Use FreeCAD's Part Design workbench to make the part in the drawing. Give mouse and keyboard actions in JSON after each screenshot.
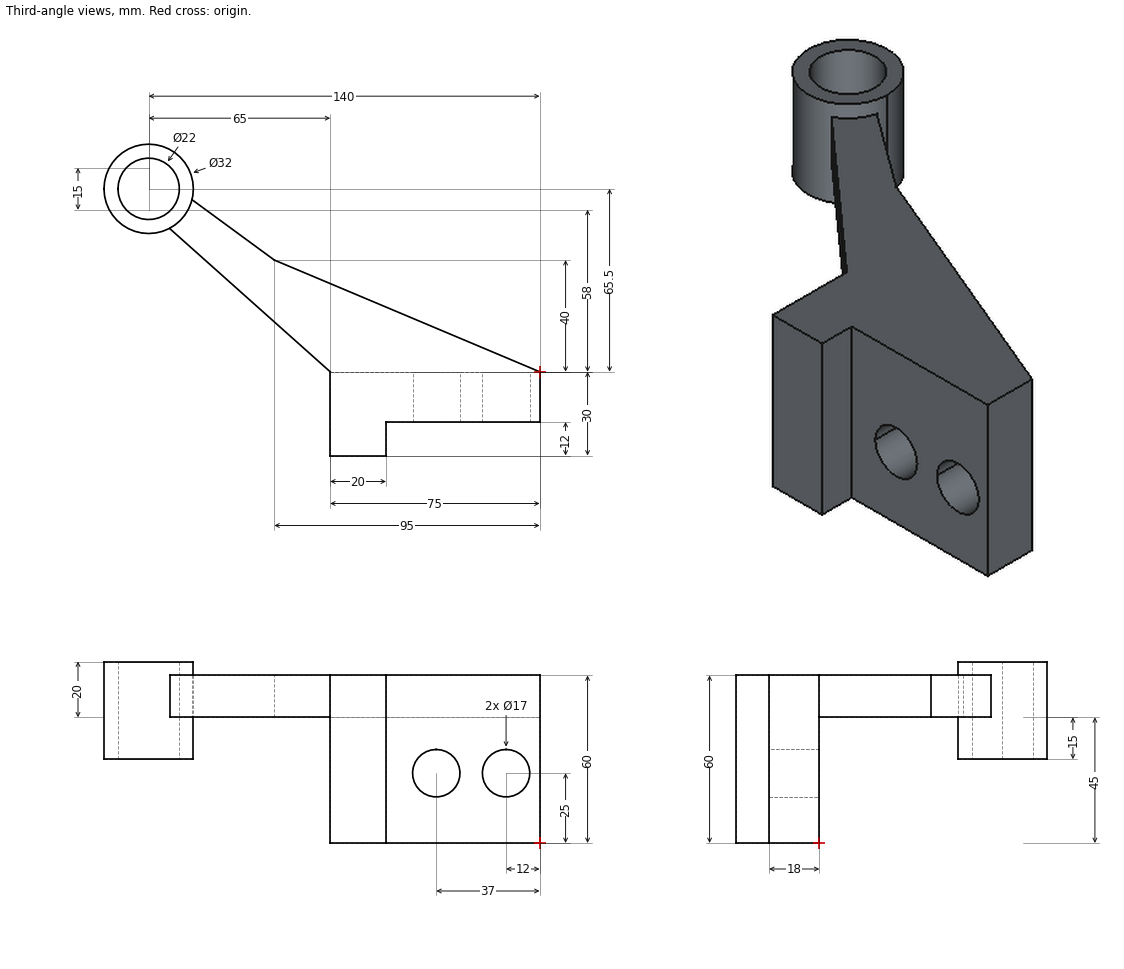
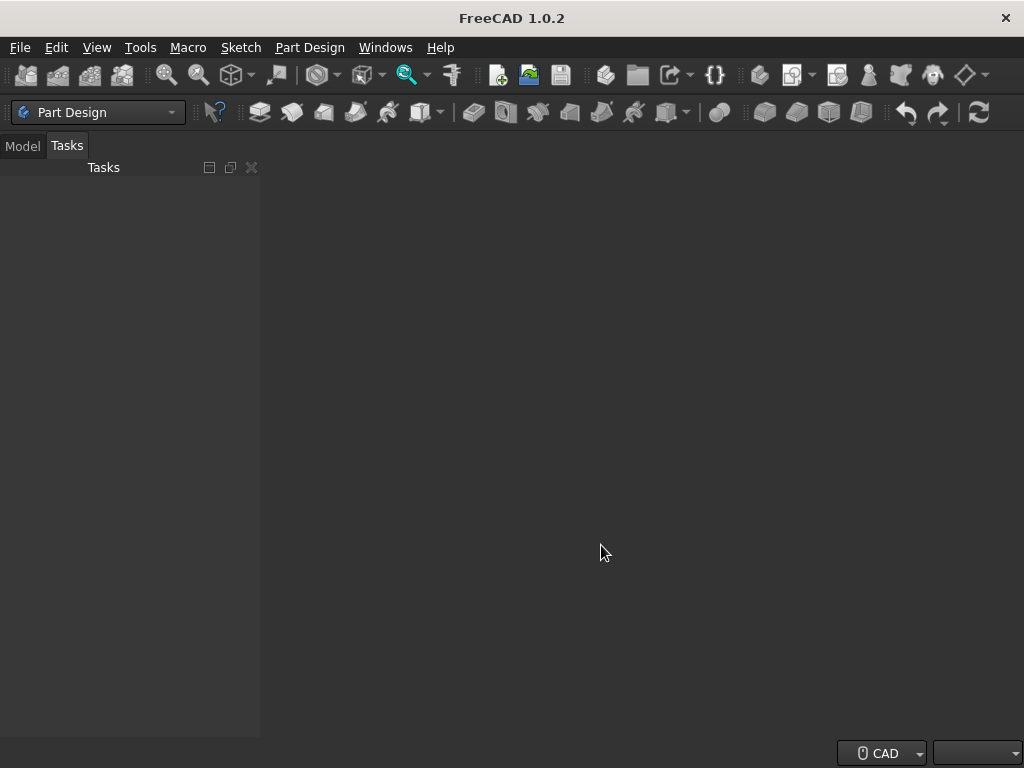
{"action": "left_click", "coordinate": [498, 76]}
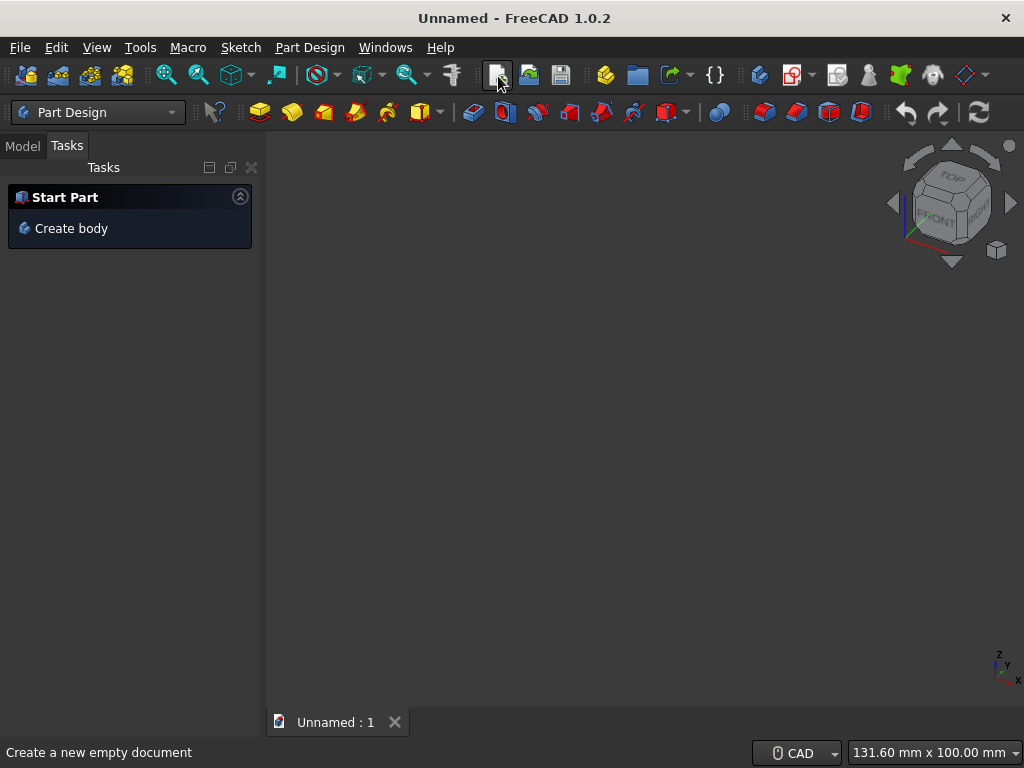
{"action": "left_click", "coordinate": [792, 76]}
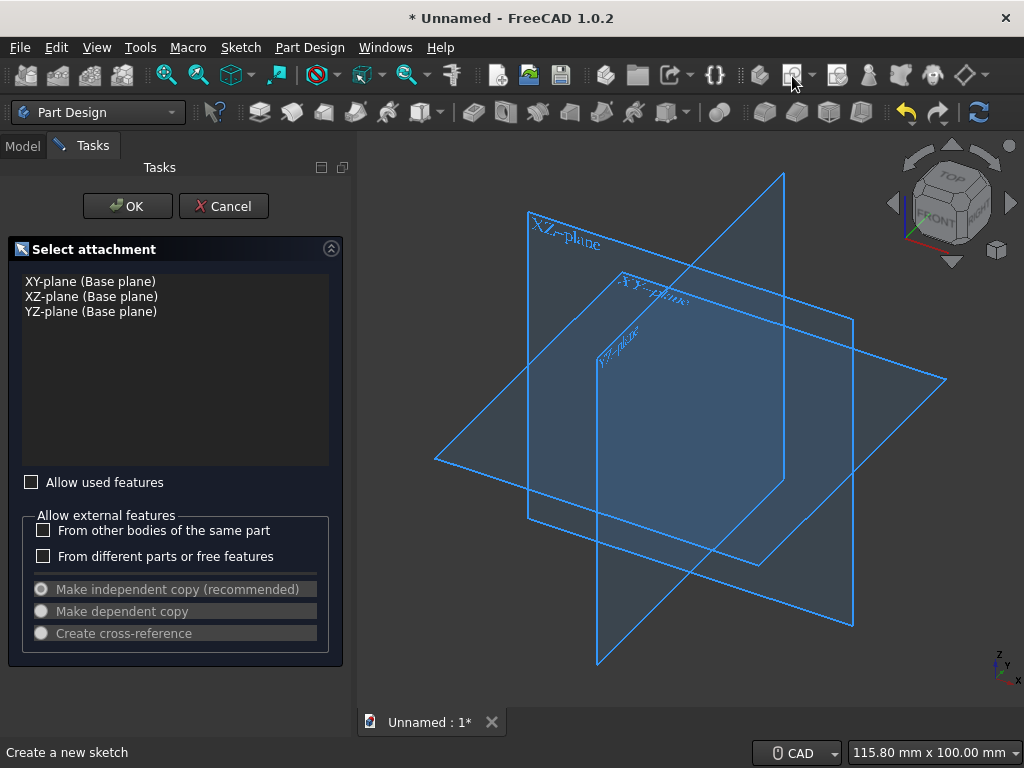
{"action": "left_click", "coordinate": [82, 282]}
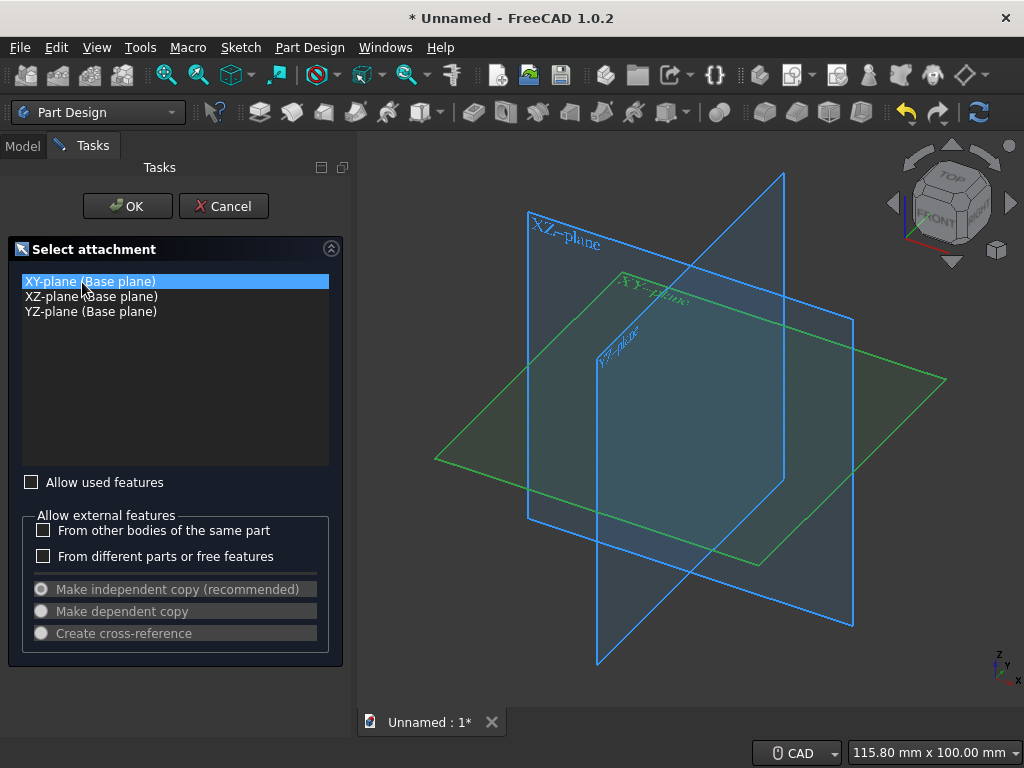
{"action": "left_click", "coordinate": [128, 206]}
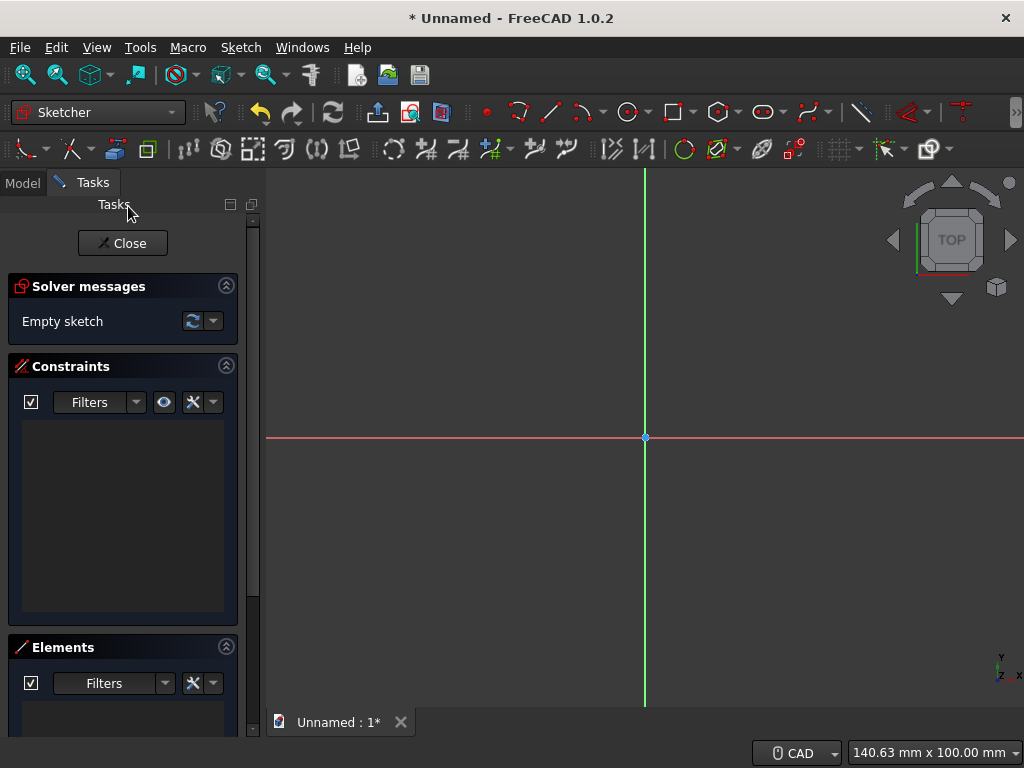
{"action": "scroll", "coordinate": [859, 196], "scroll_direction": "down", "scroll_amount": 1}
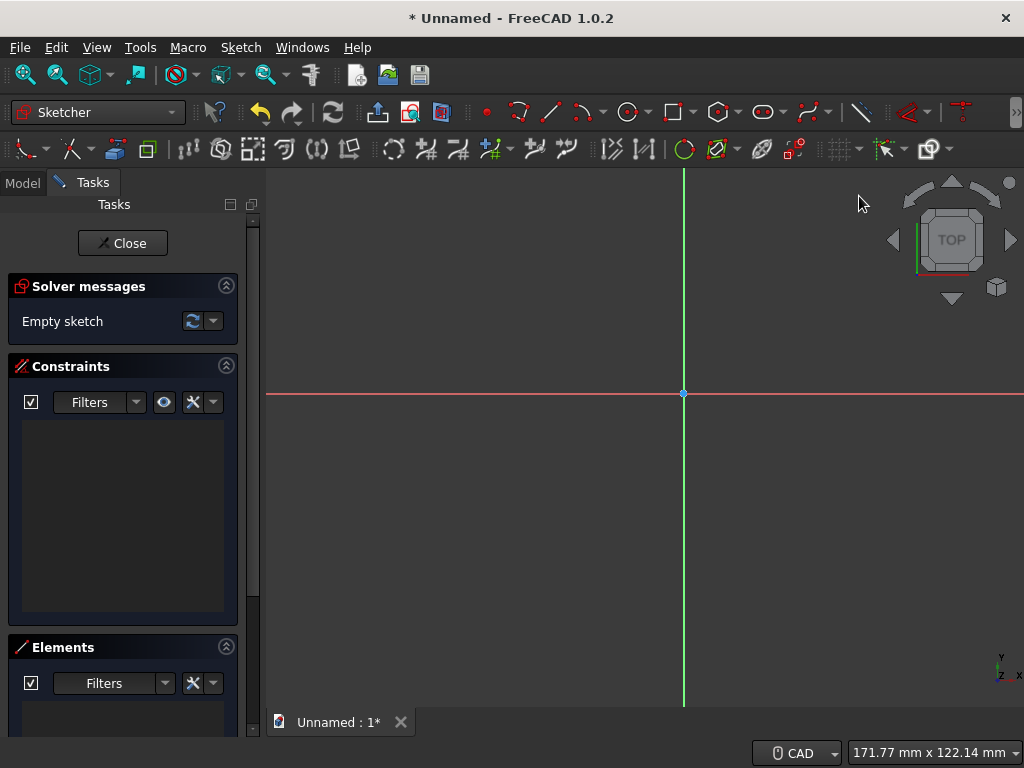
{"action": "left_click", "coordinate": [520, 112]}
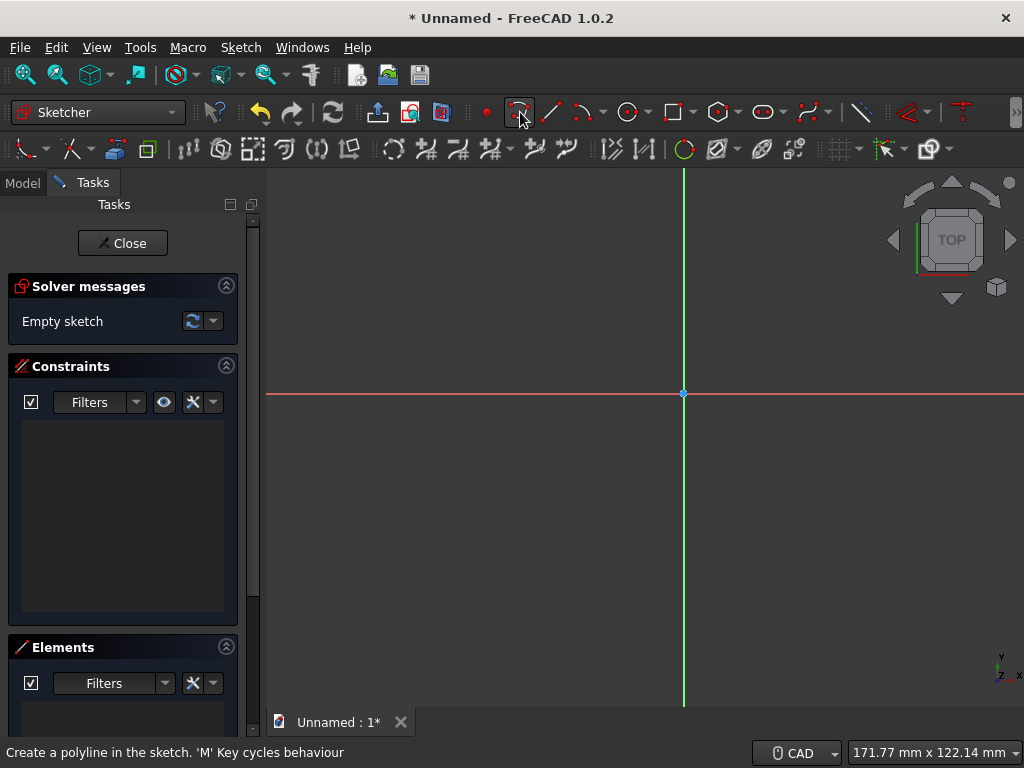
{"action": "left_click", "coordinate": [684, 394]}
{"action": "left_click", "coordinate": [353, 403]}
{"action": "left_click", "coordinate": [353, 526]}
{"action": "left_click", "coordinate": [441, 526]}
{"action": "left_click", "coordinate": [441, 473]}
{"action": "left_click", "coordinate": [675, 473]}
{"action": "left_click", "coordinate": [684, 394]}
{"action": "key", "text": "Escape"}
{"action": "key", "text": "Escape"}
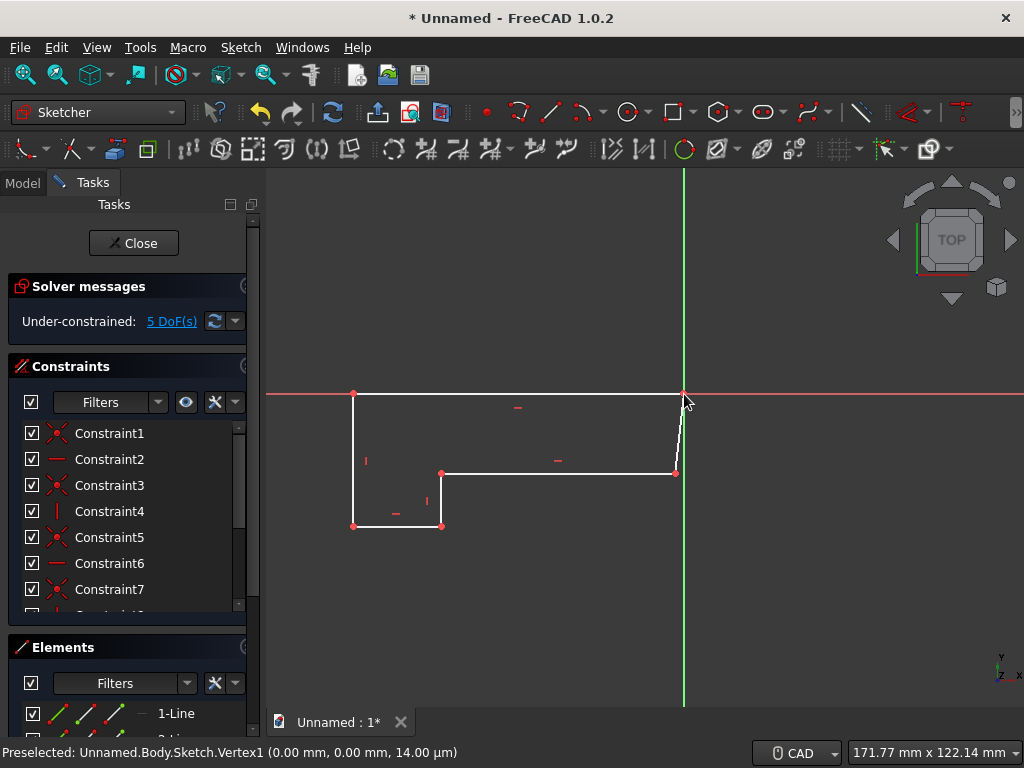
{"action": "left_click", "coordinate": [681, 418]}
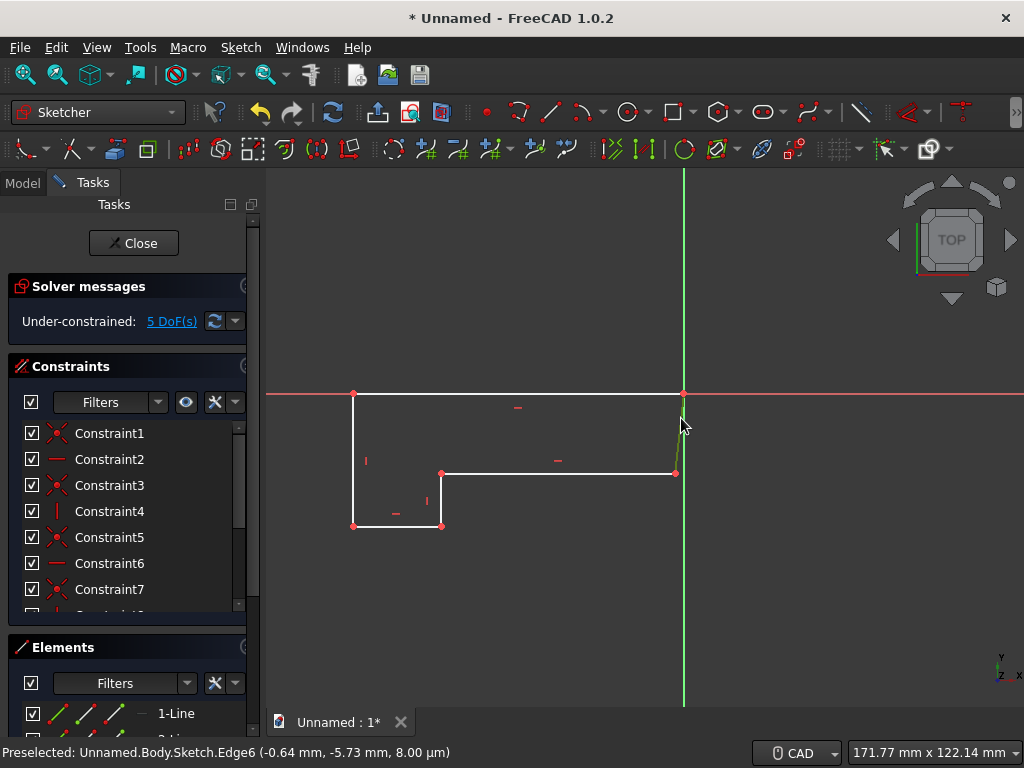
{"action": "key", "text": "v"}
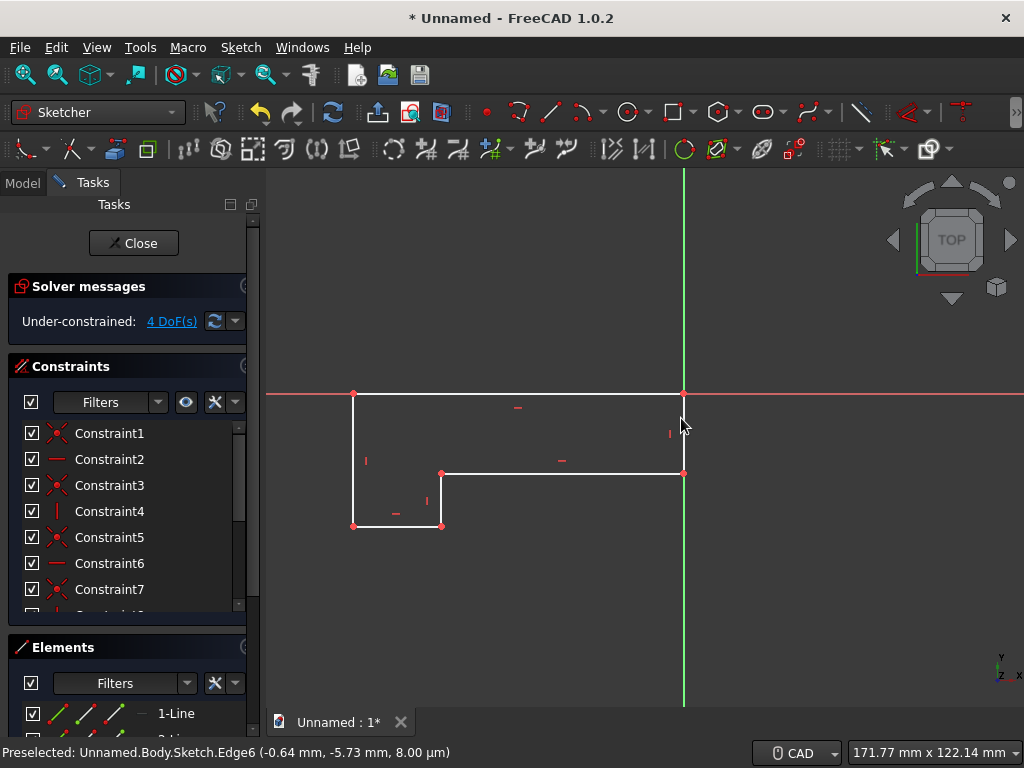
{"action": "left_click", "coordinate": [585, 394]}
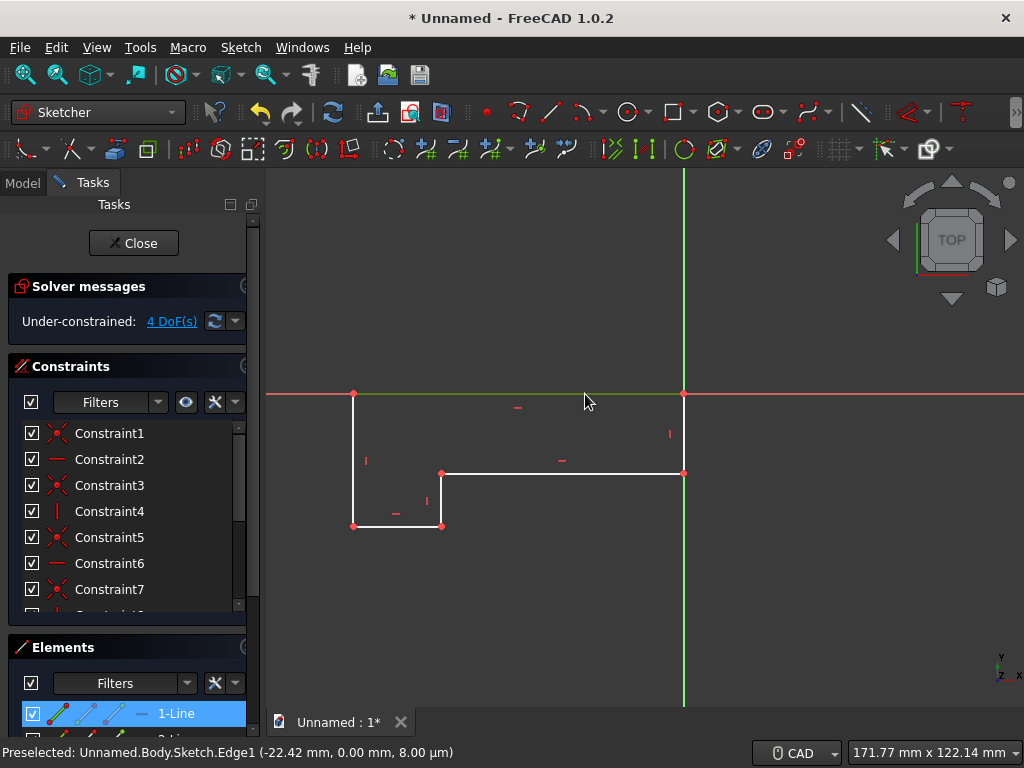
{"action": "key", "text": "l"}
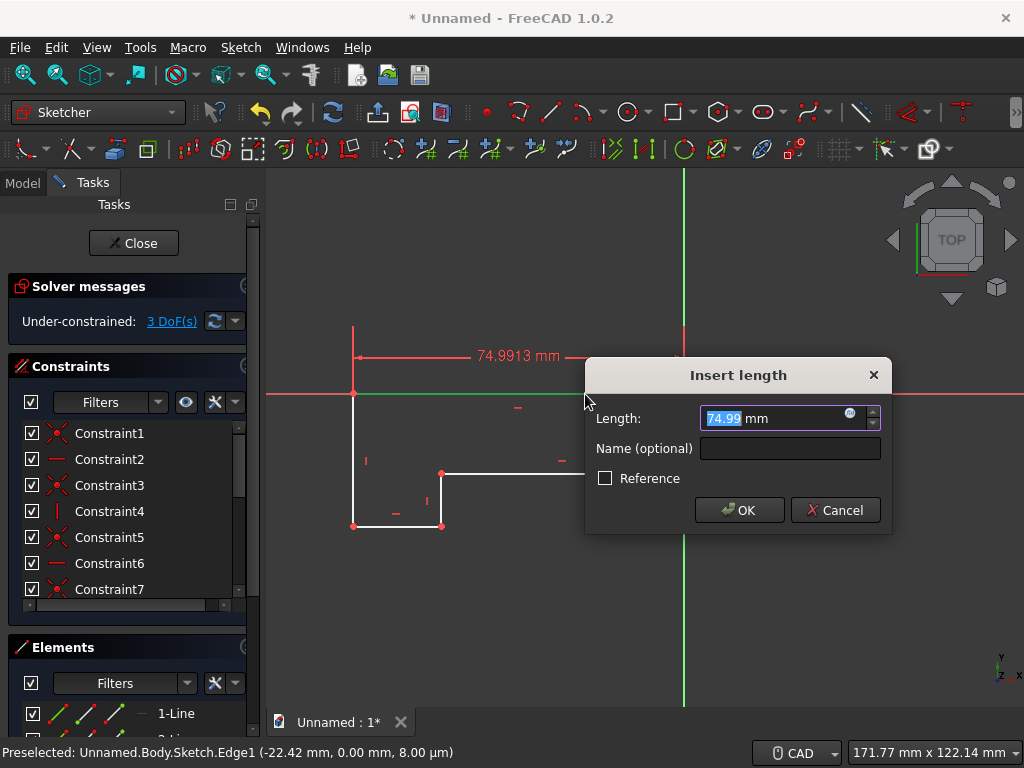
{"action": "type", "text": "75"}
{"action": "key", "text": "Return"}